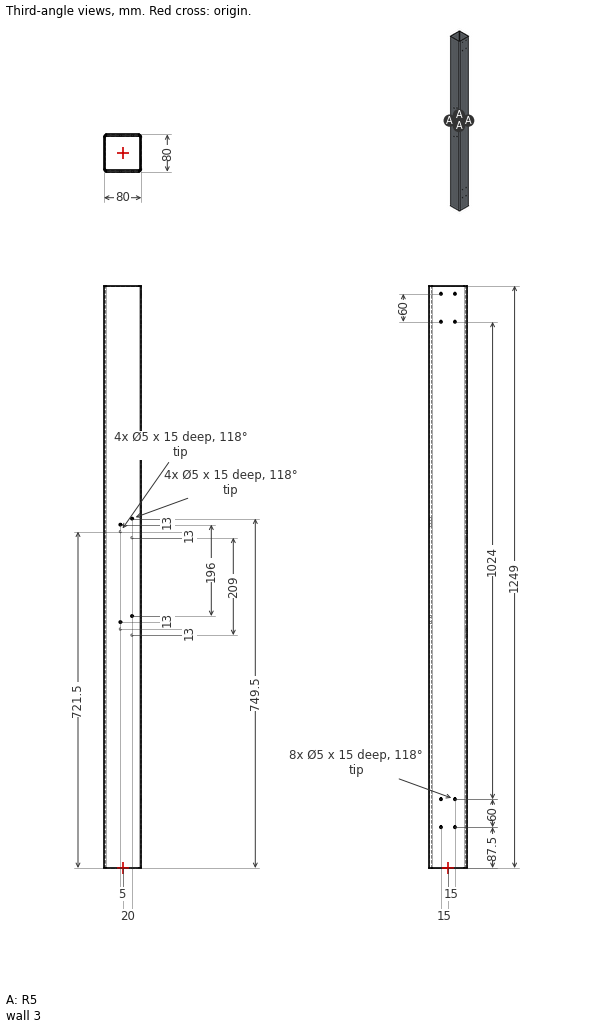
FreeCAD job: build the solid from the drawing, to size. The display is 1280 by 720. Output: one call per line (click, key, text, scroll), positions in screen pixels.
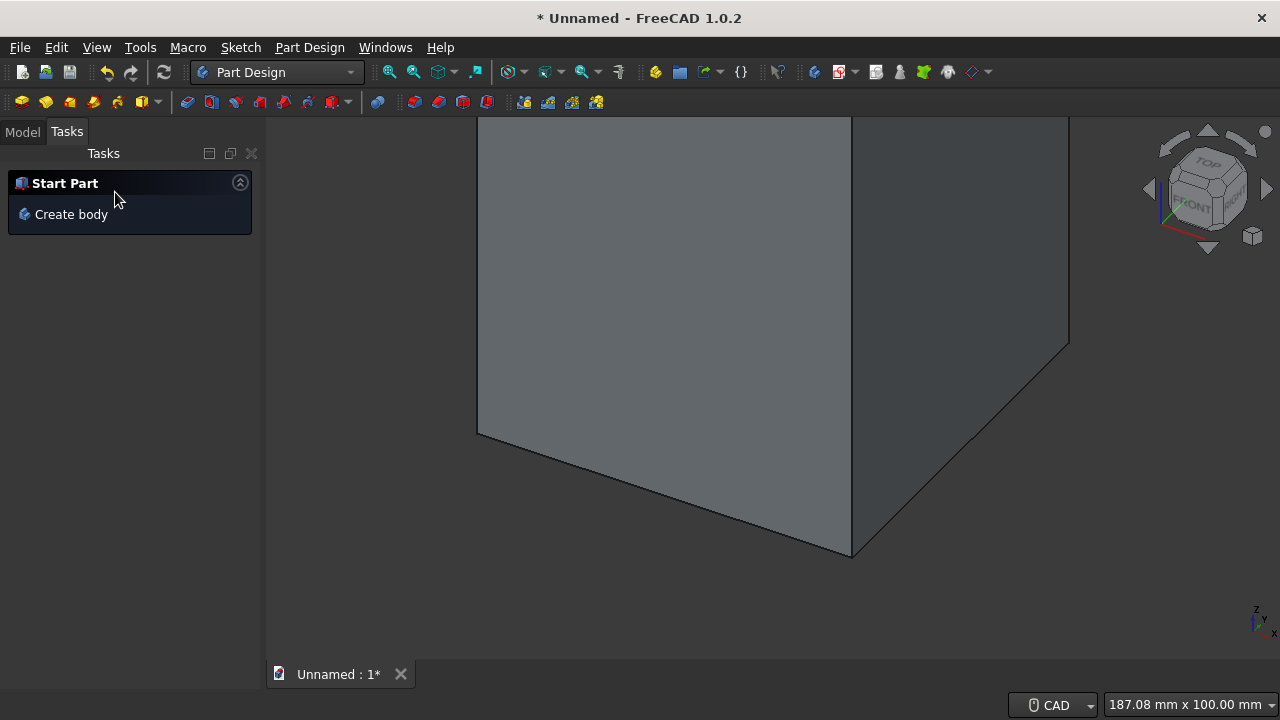
key(v)
key(f)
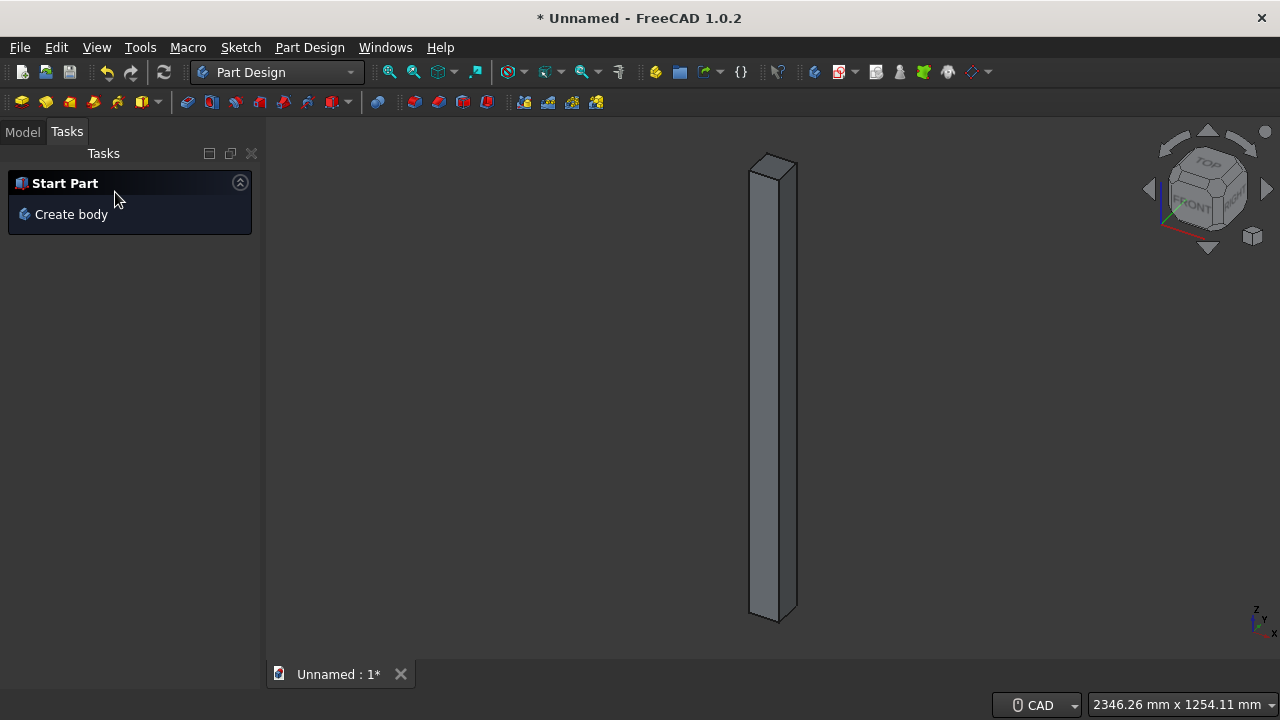
click(779, 401)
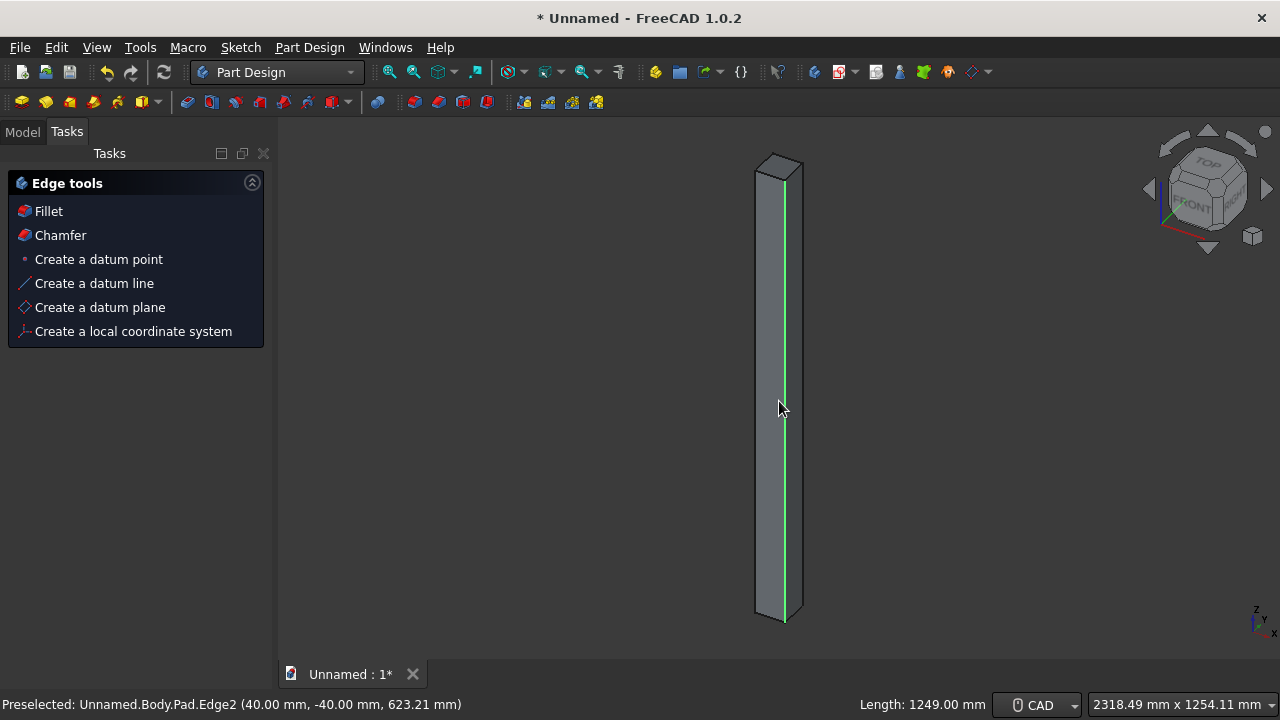
key(0)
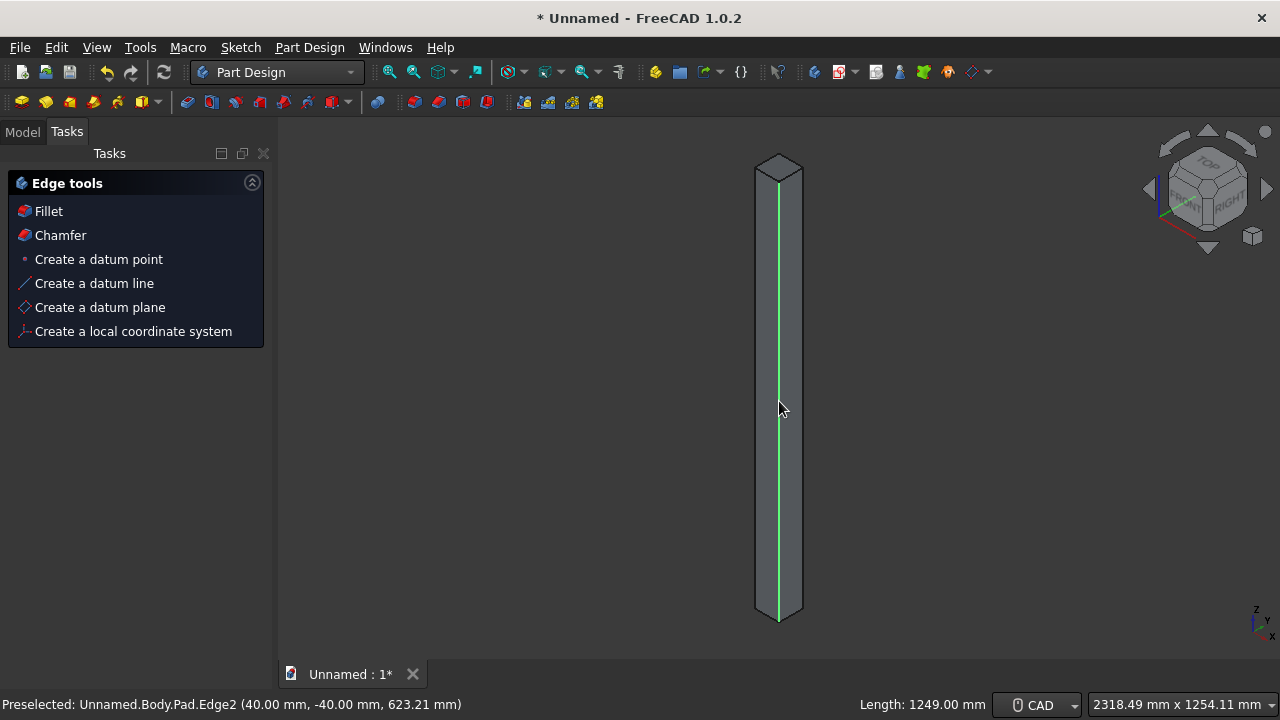
key(2)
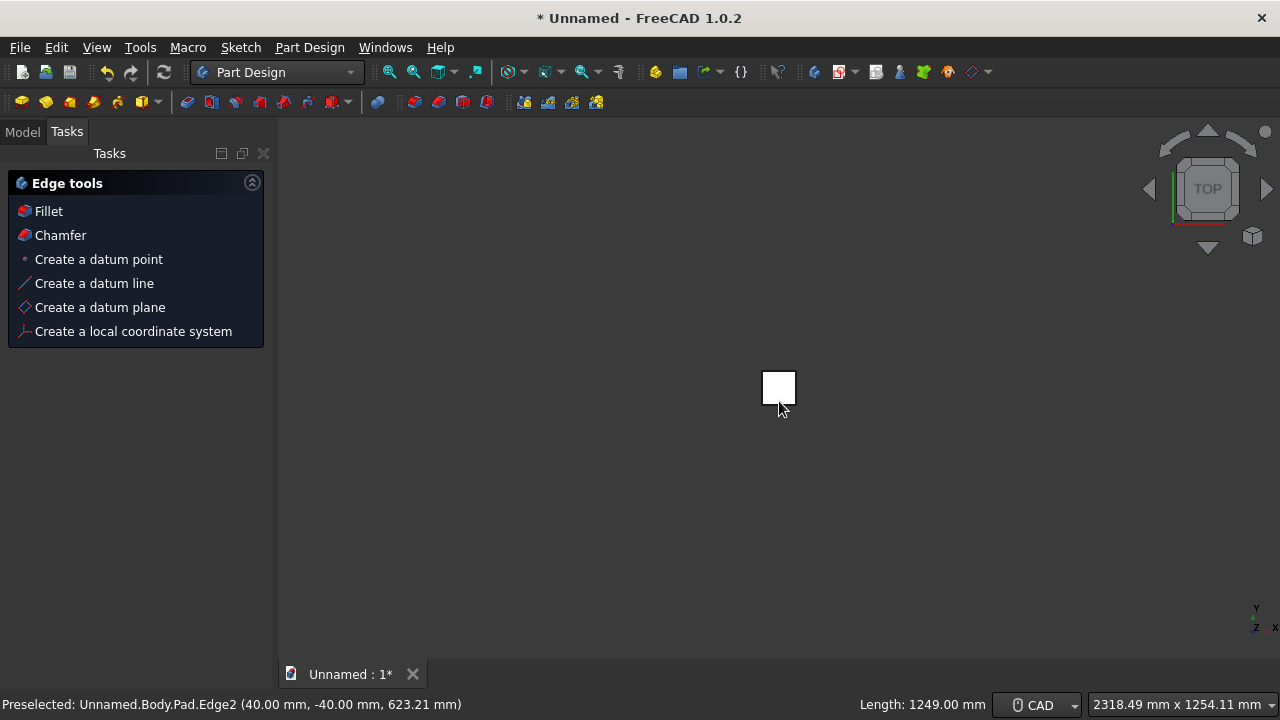
click(390, 72)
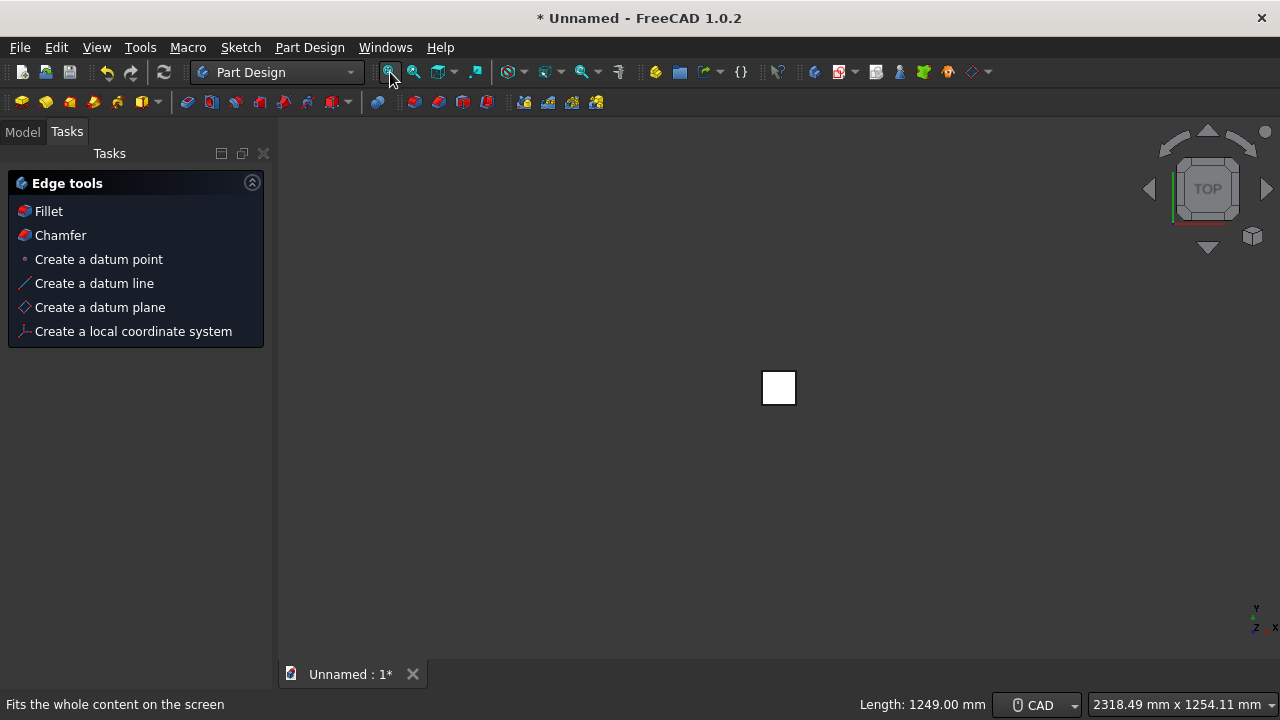
key(1)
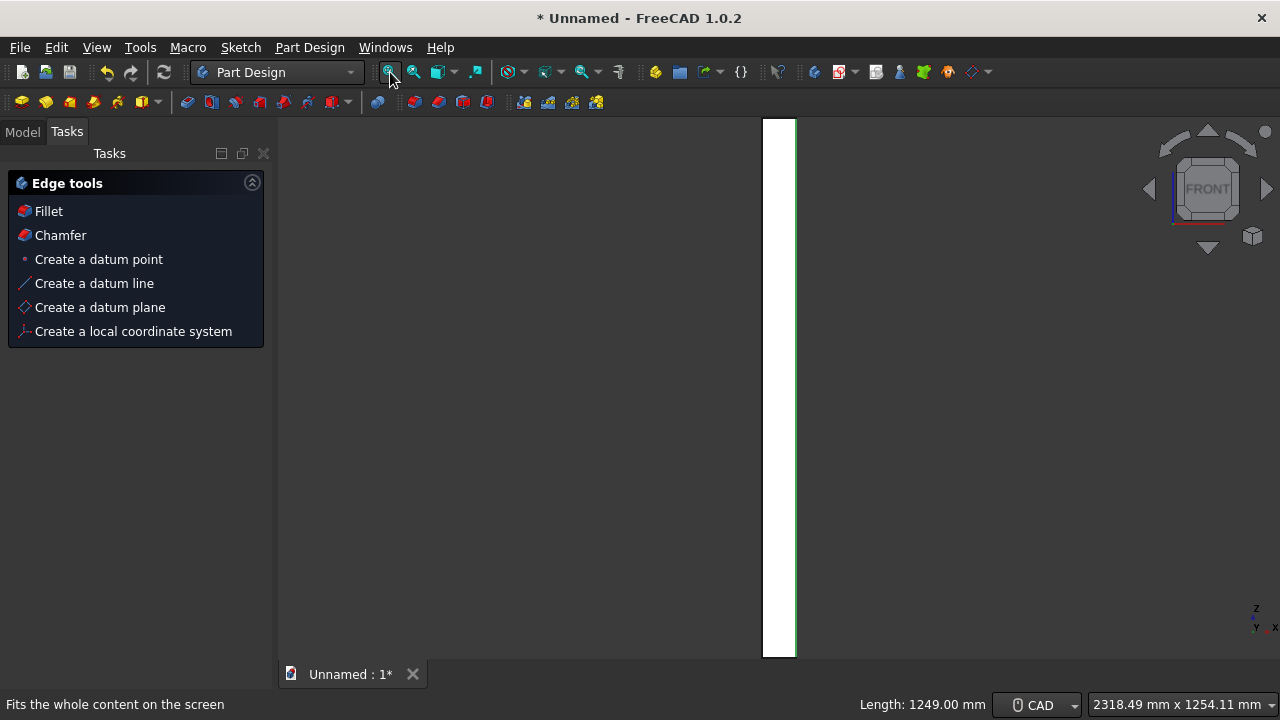
click(762, 387, ctrl)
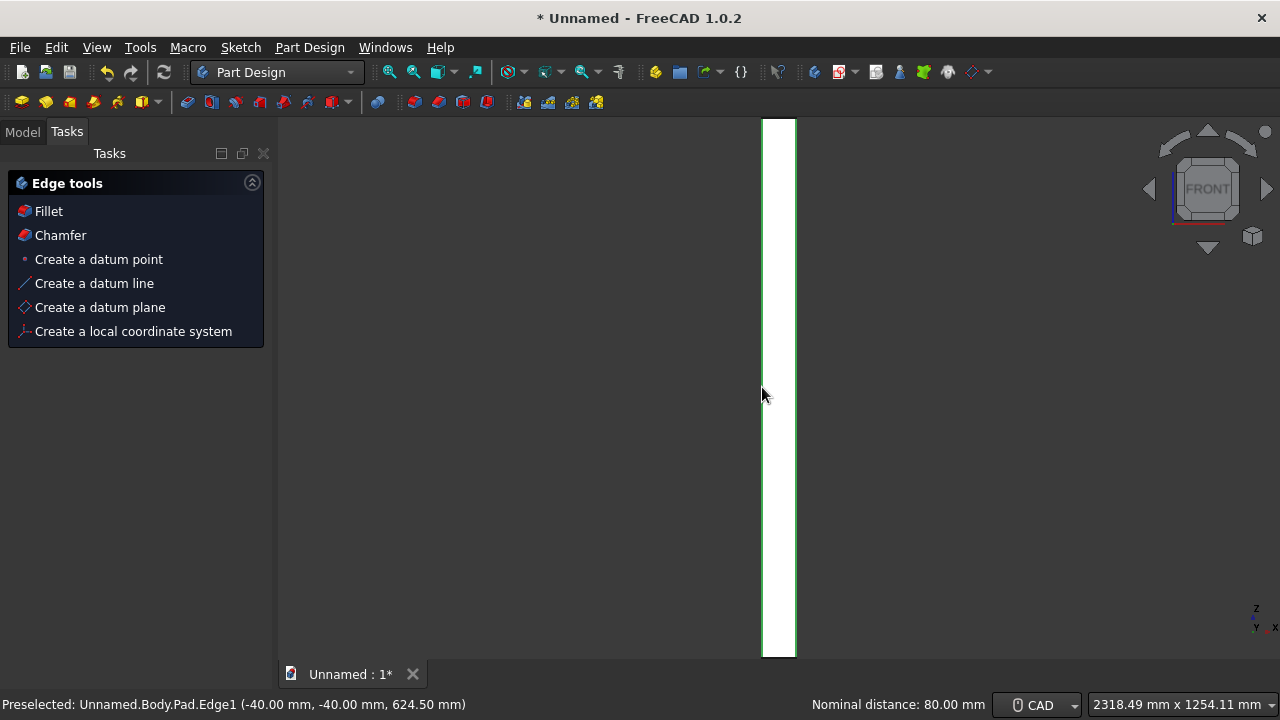
key(3)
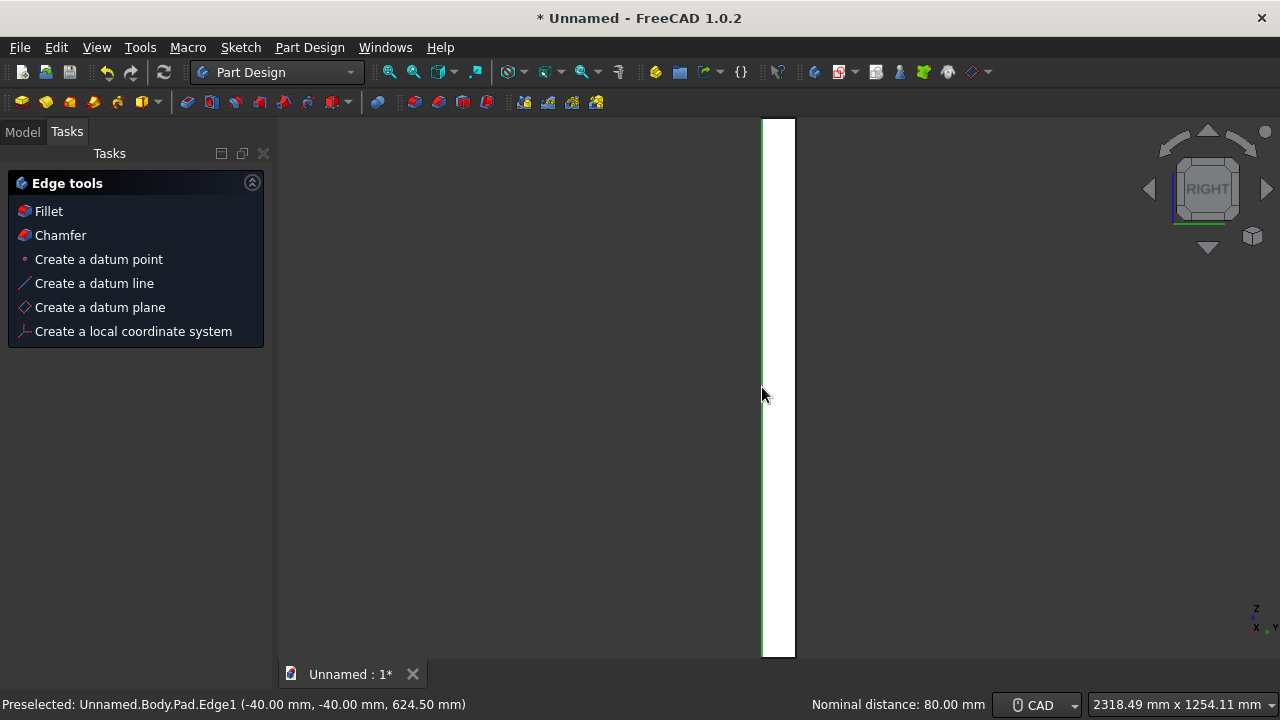
click(796, 387, ctrl)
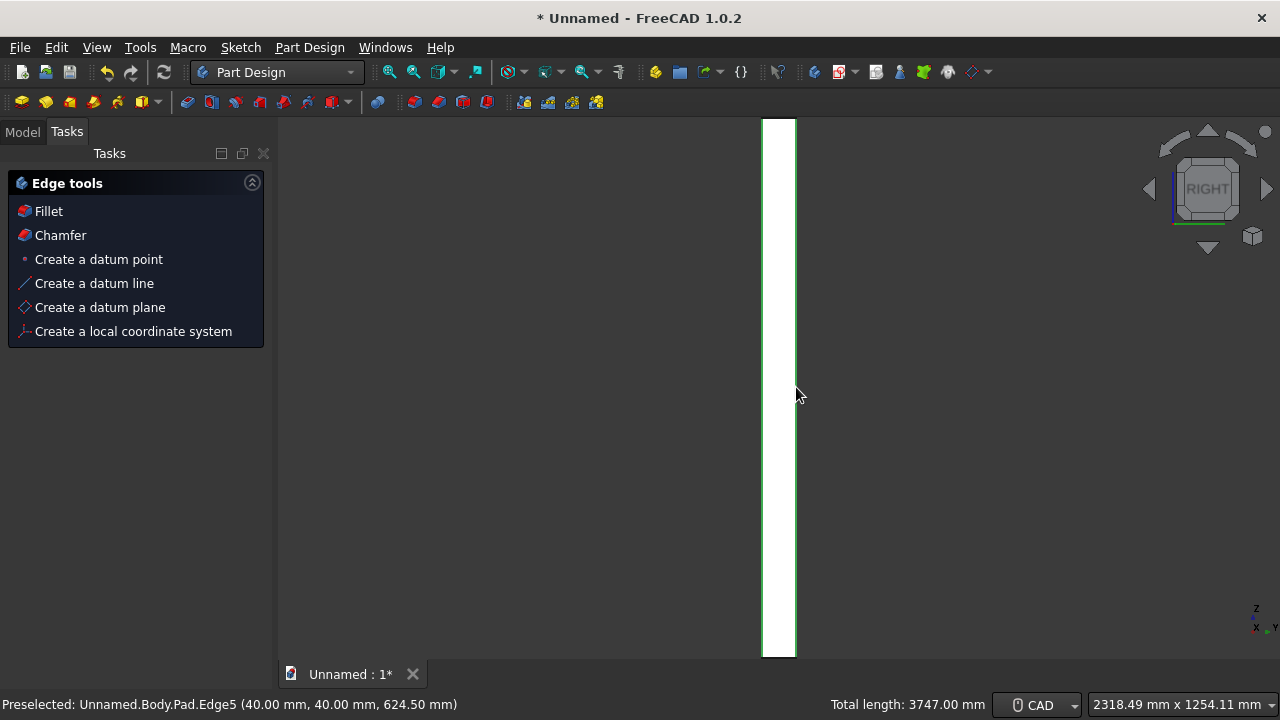
key(5)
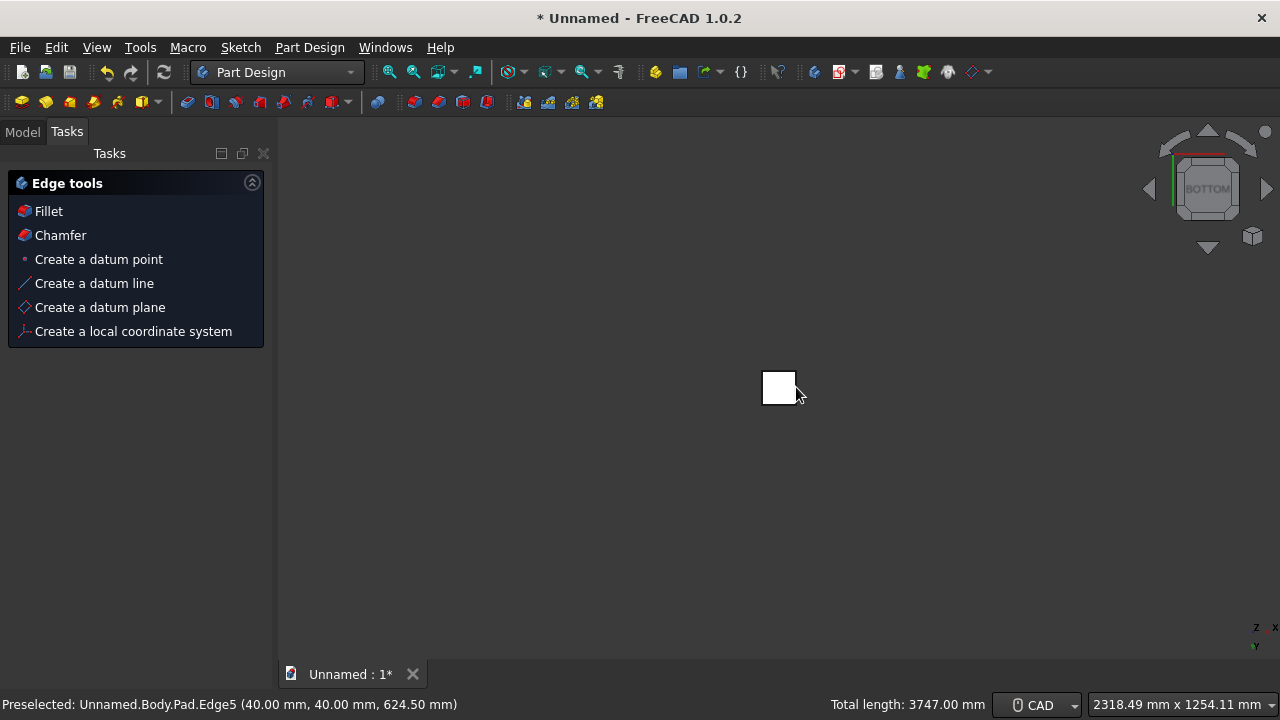
key(v)
key(f)